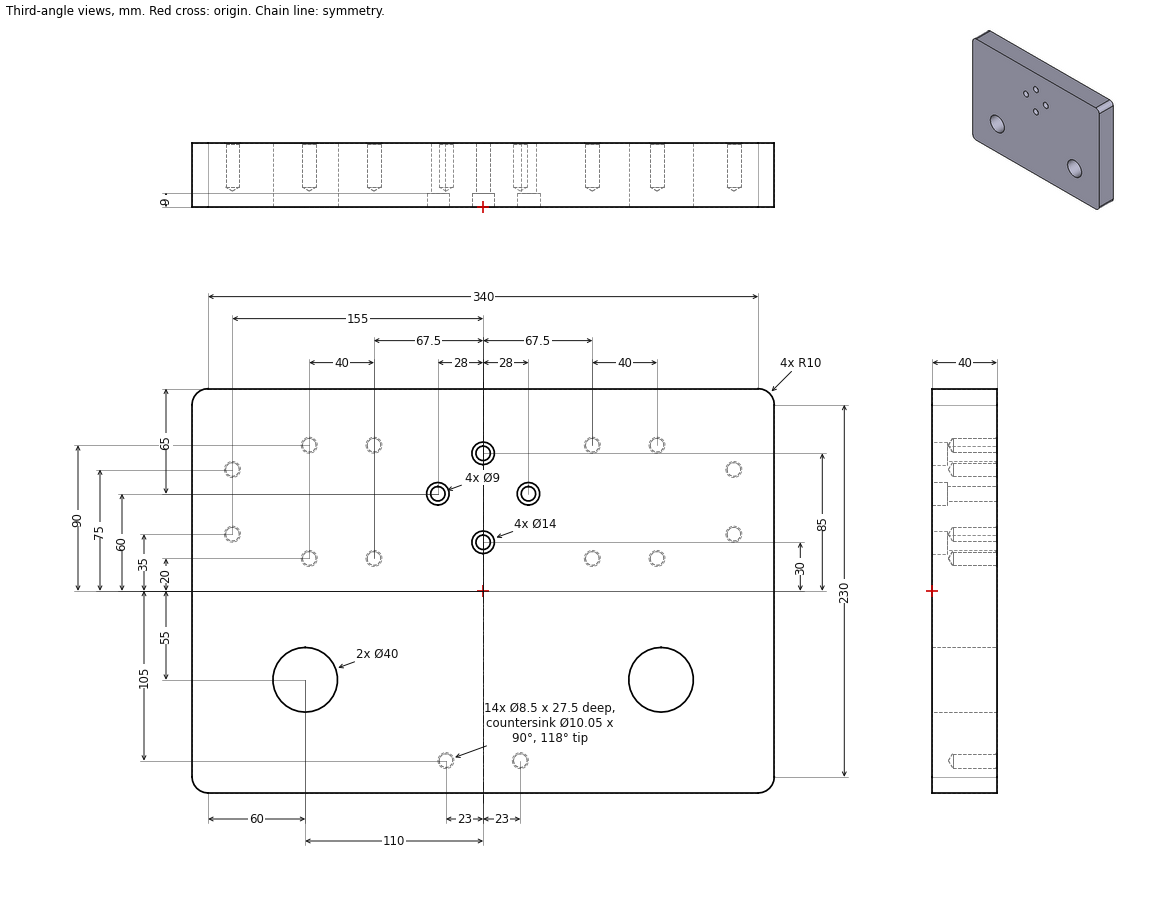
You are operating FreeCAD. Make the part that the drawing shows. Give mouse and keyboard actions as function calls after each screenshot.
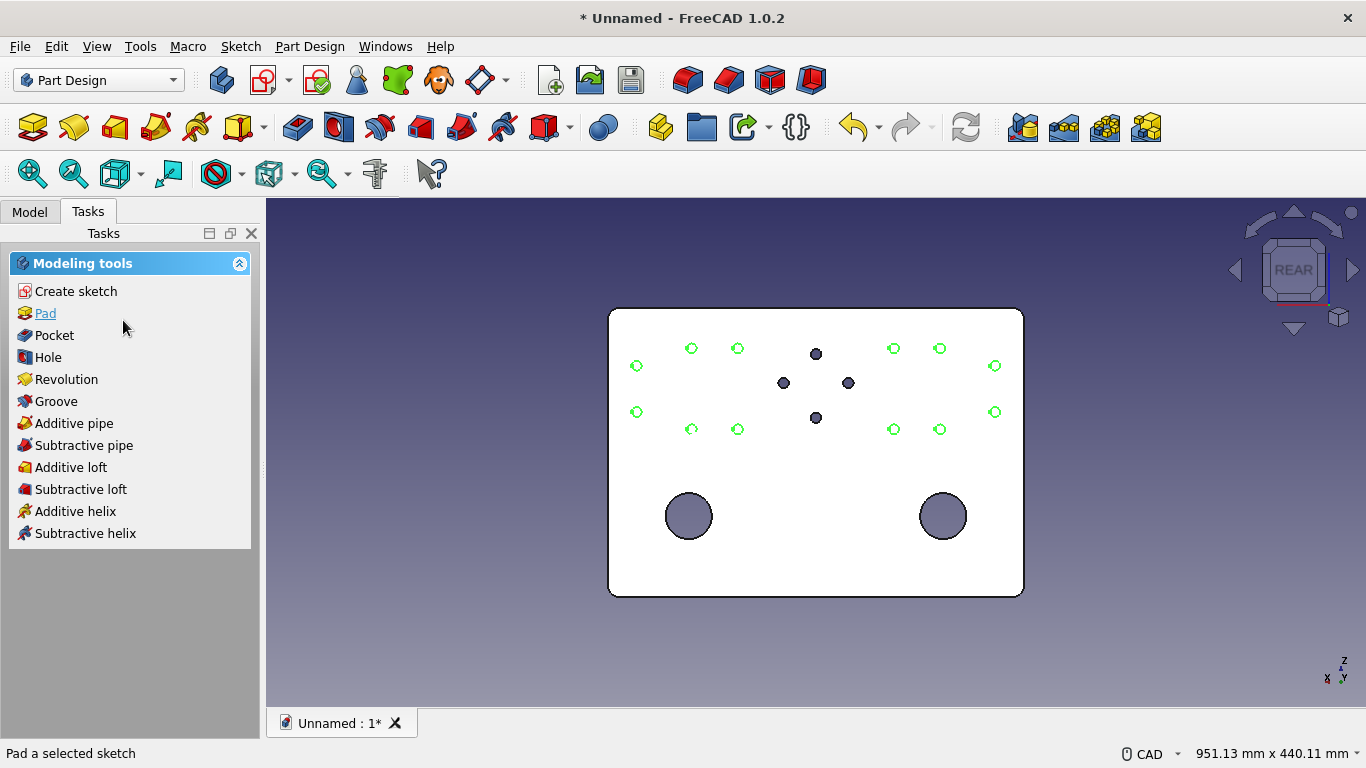
click(339, 128)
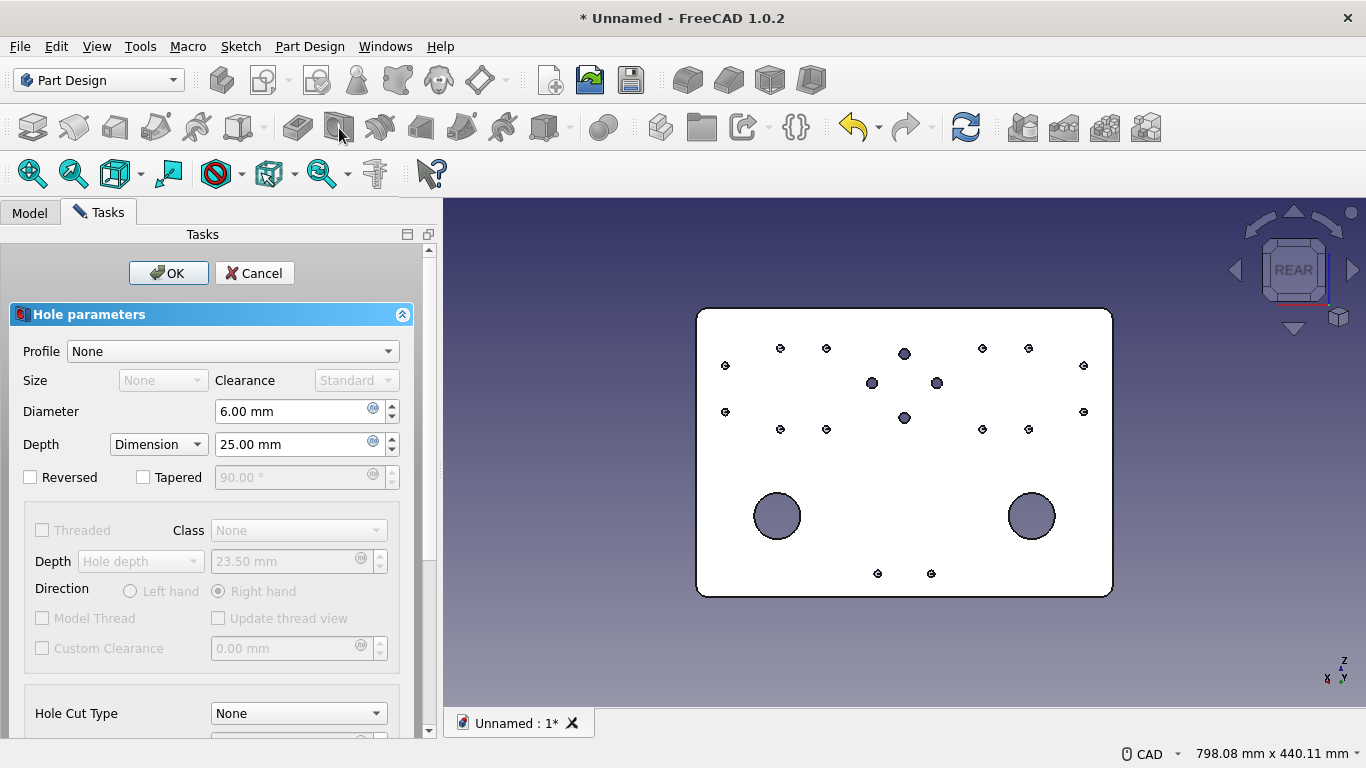
triple_click(300, 412)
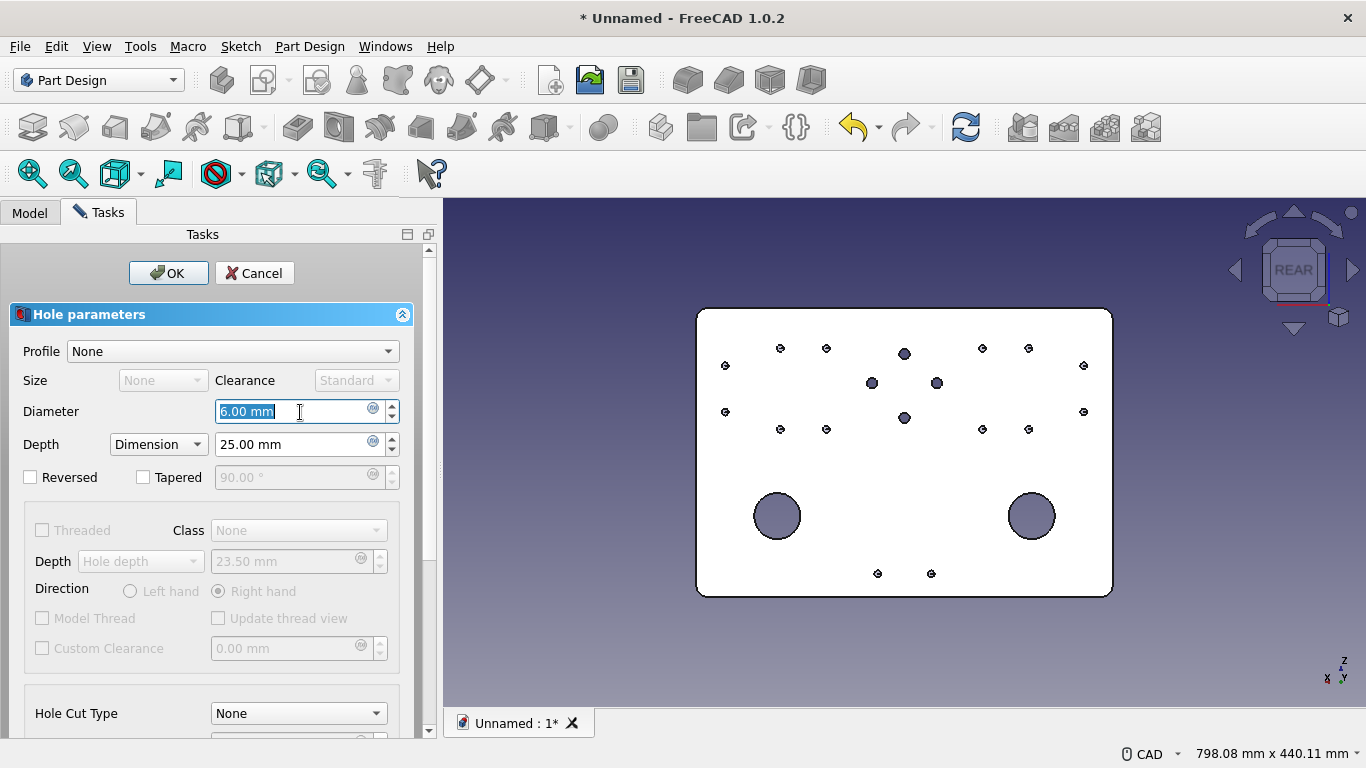
text(8.5)
key(Tab)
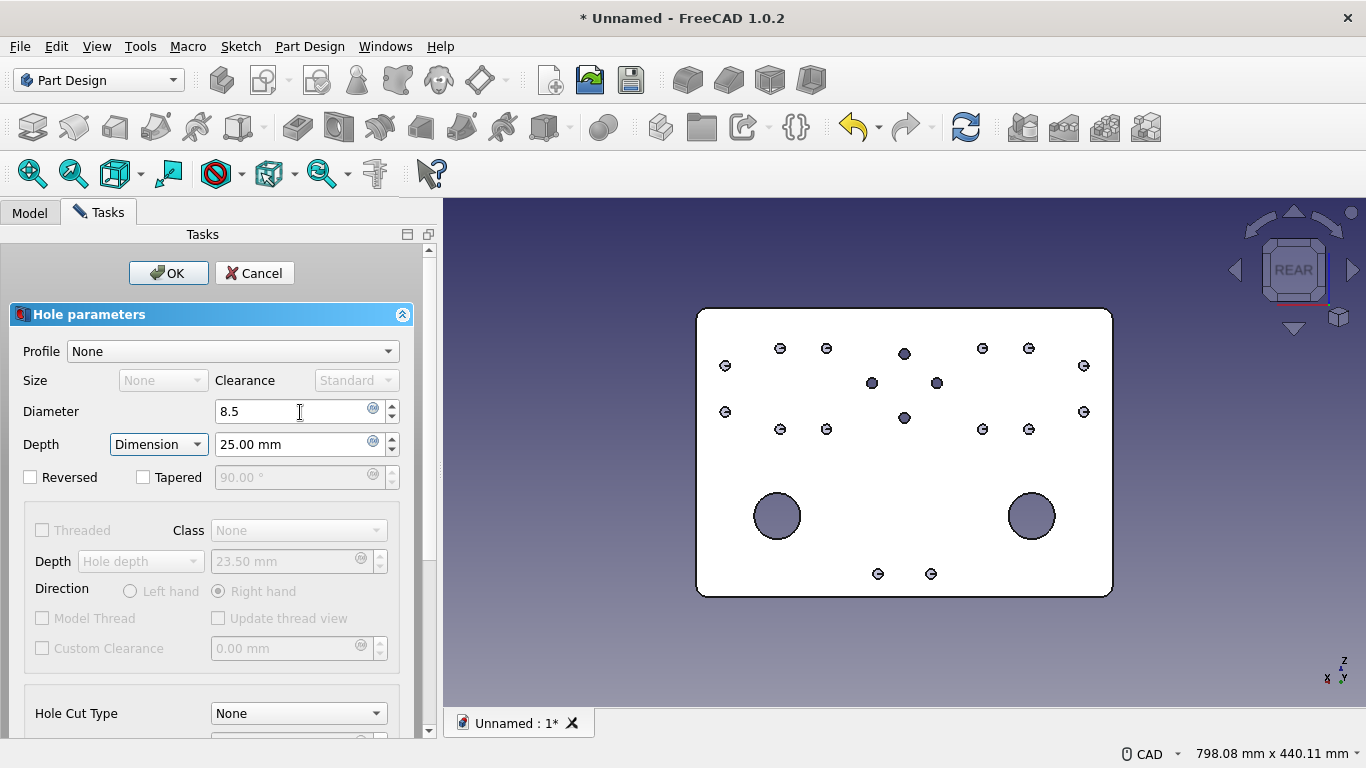
triple_click(300, 444)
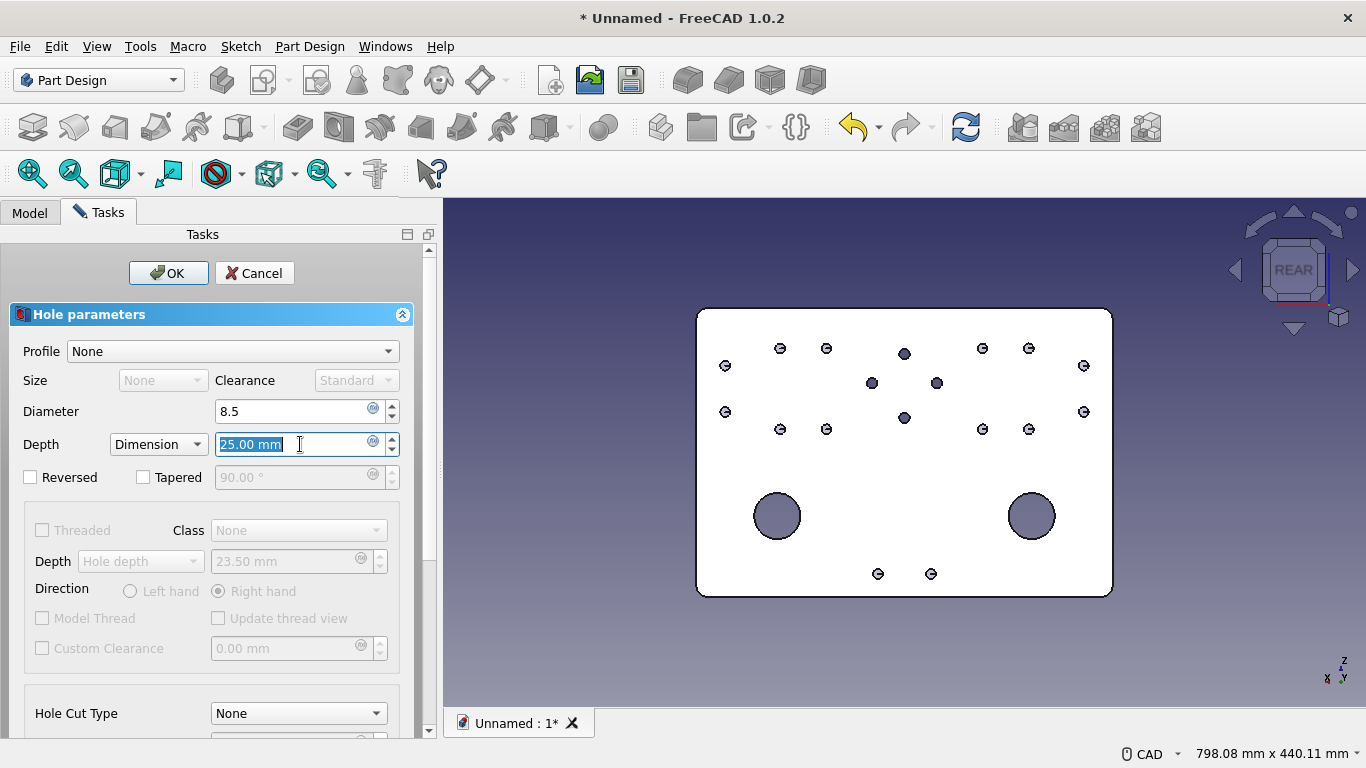
text(27.5)
key(Tab)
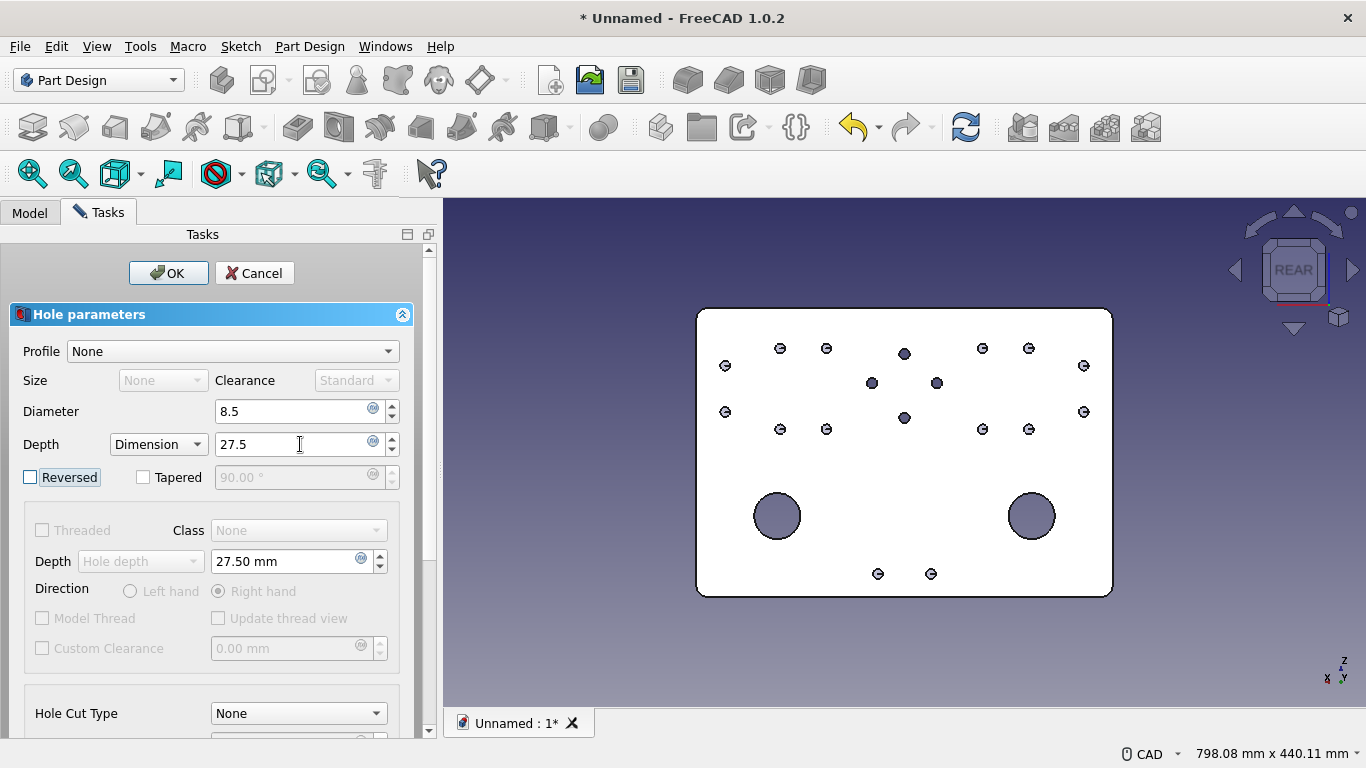
click(300, 714)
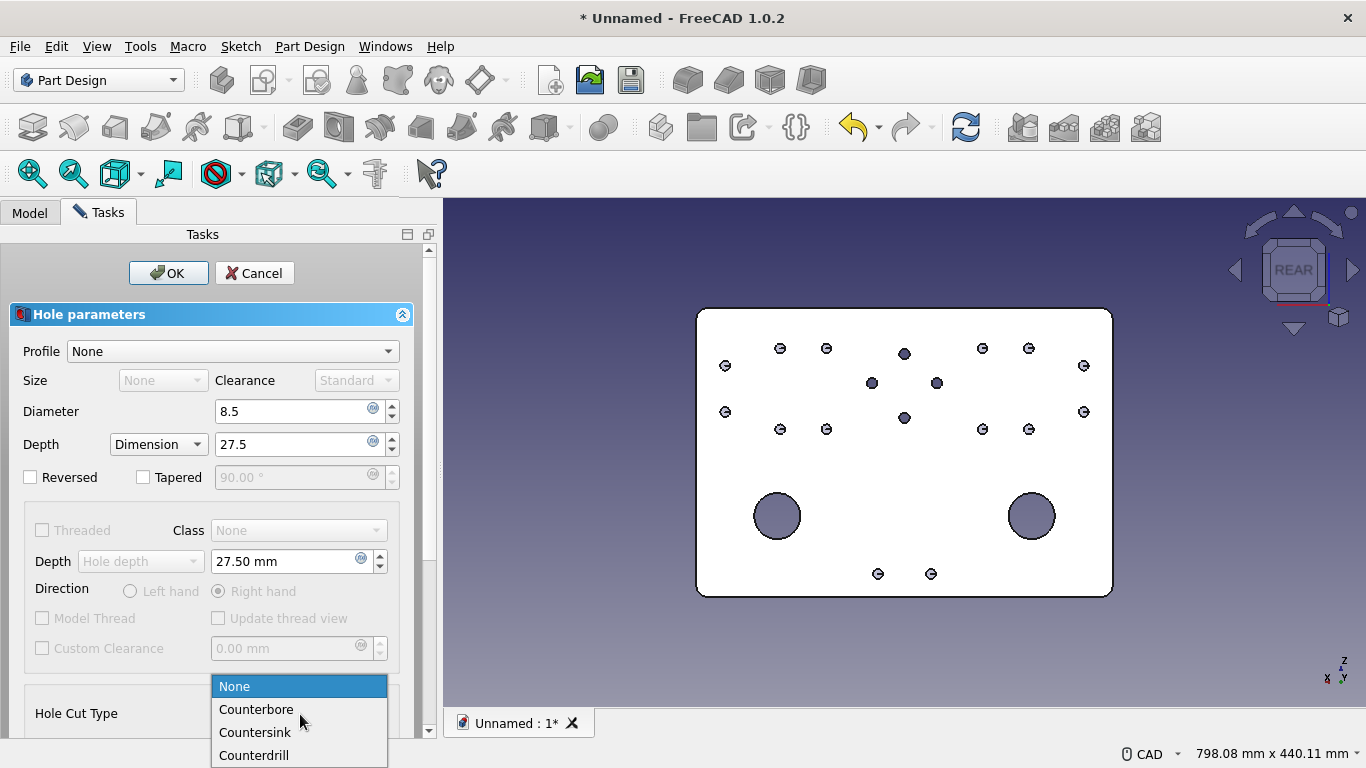
click(298, 732)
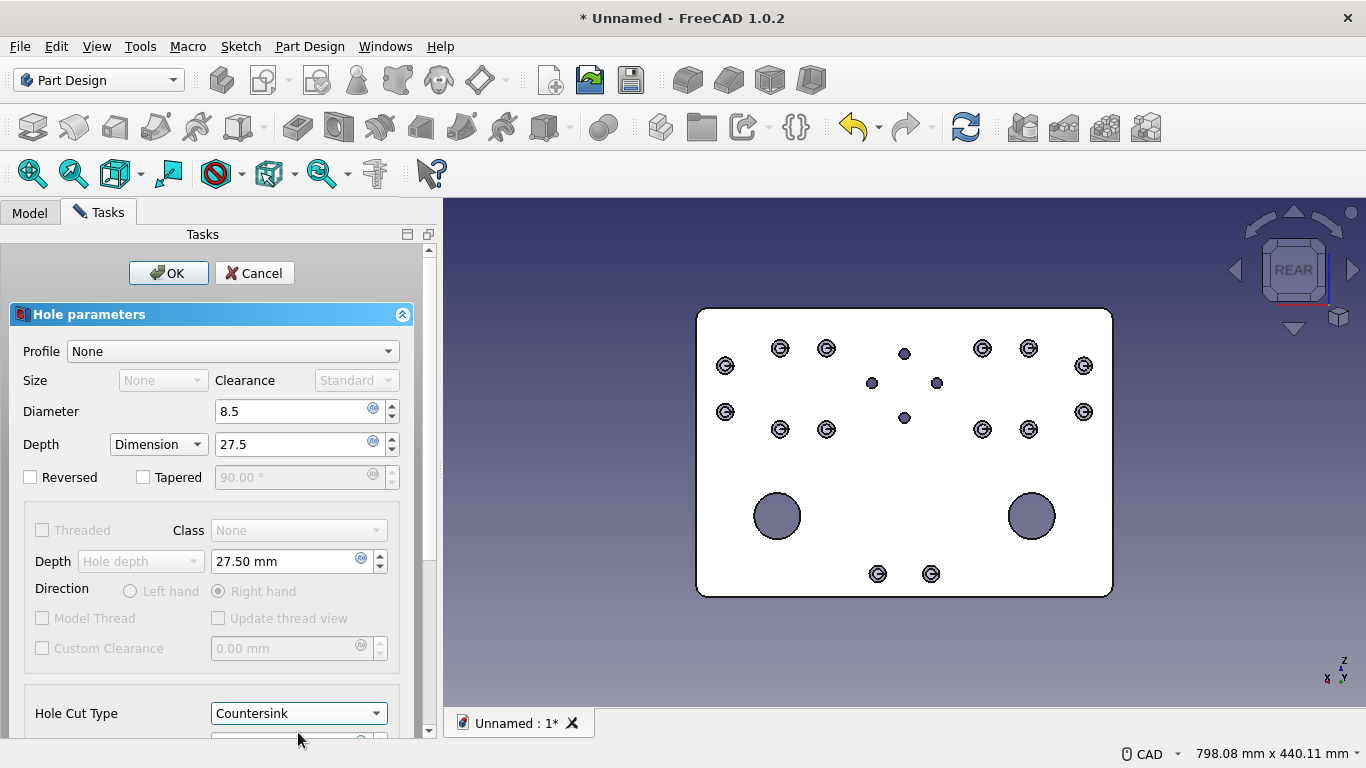
scroll(429, 491, down, 2)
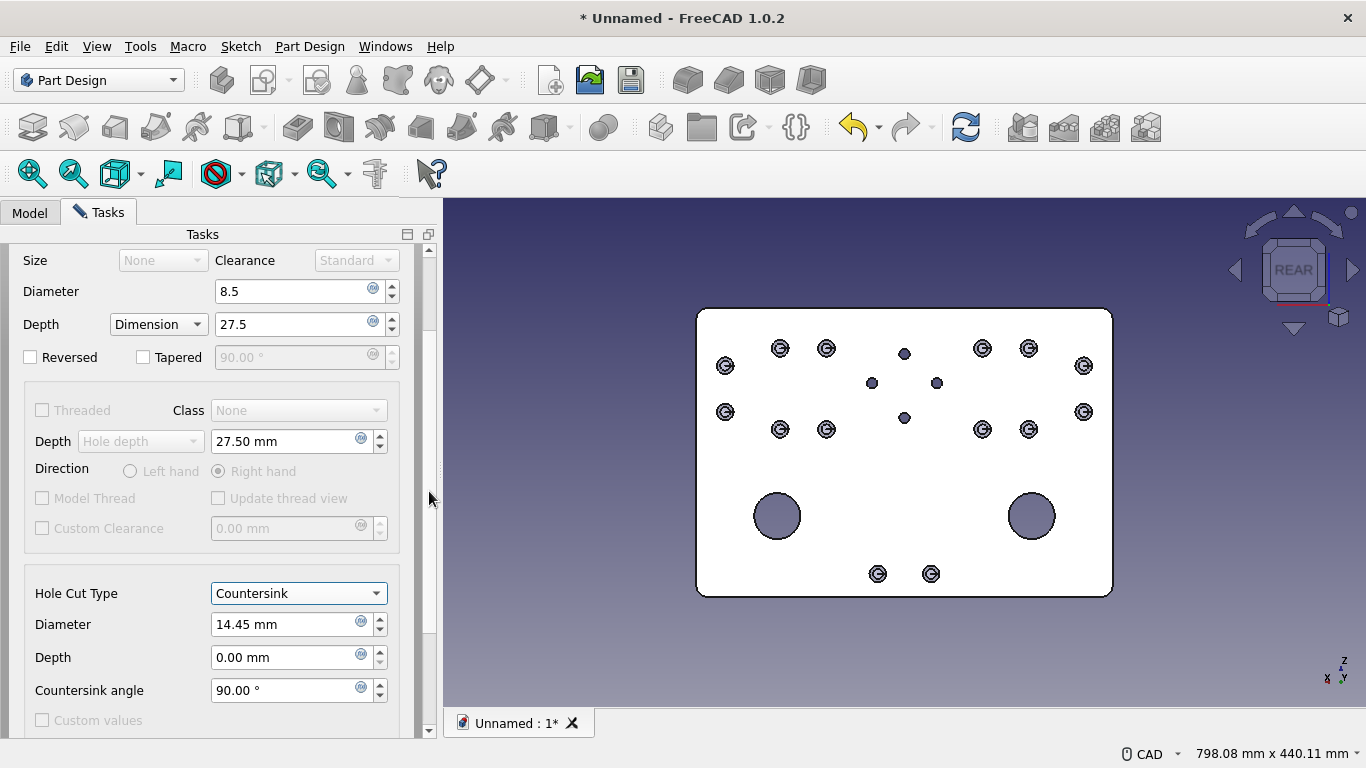
triple_click(292, 624)